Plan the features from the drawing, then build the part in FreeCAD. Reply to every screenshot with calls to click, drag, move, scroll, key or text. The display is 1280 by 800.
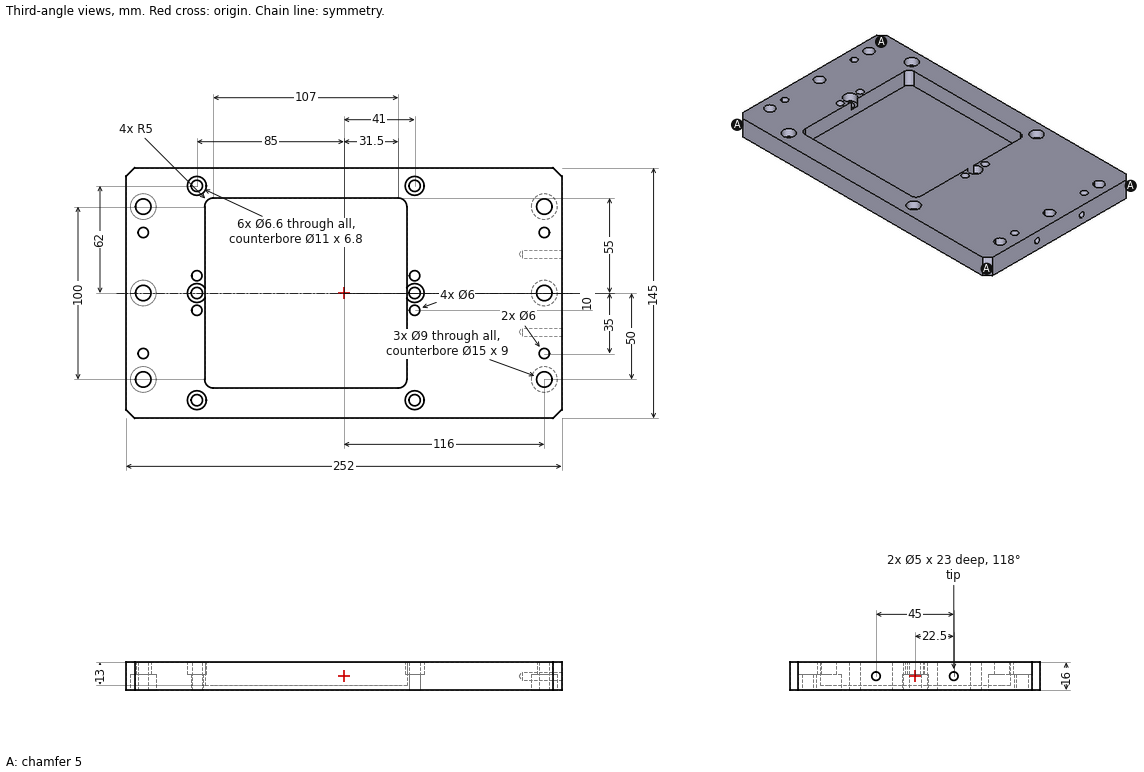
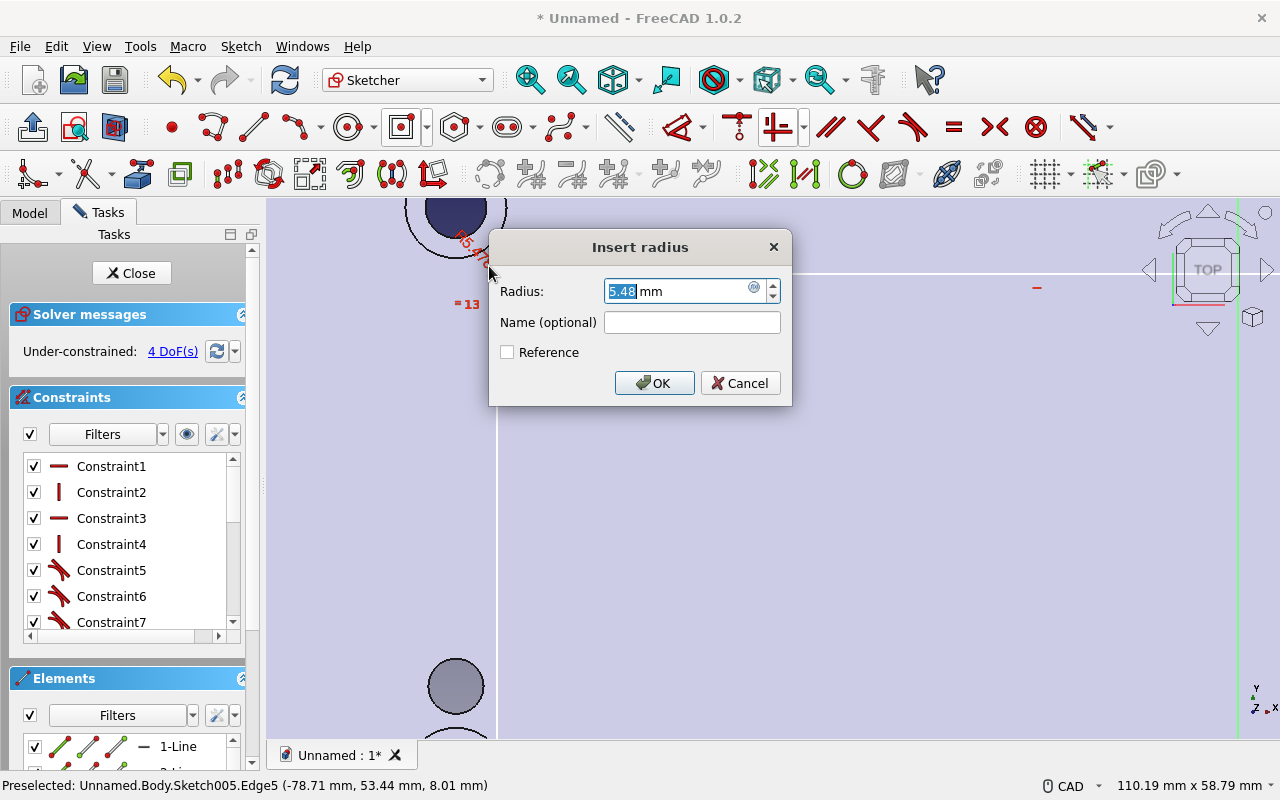
text(5)
key(Return)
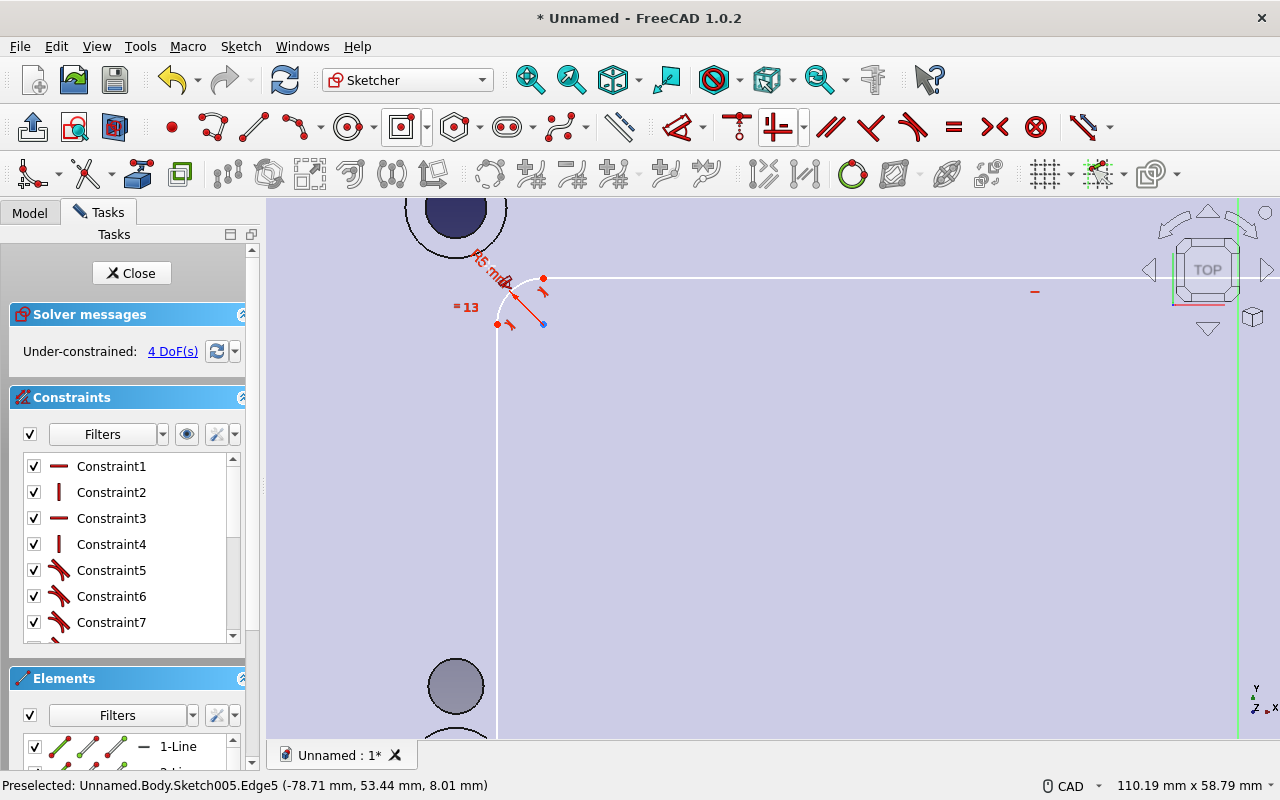
click(838, 278)
click(829, 244)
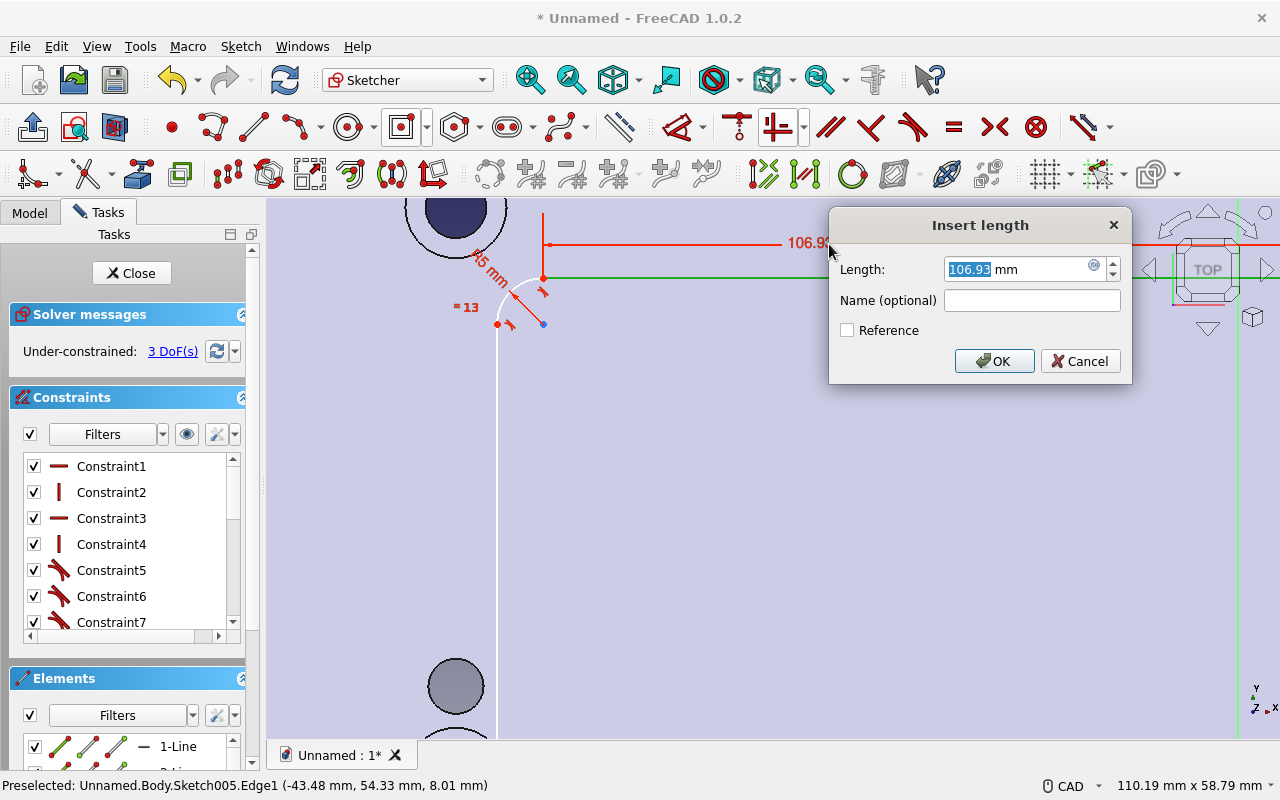
text(107)
key(Return)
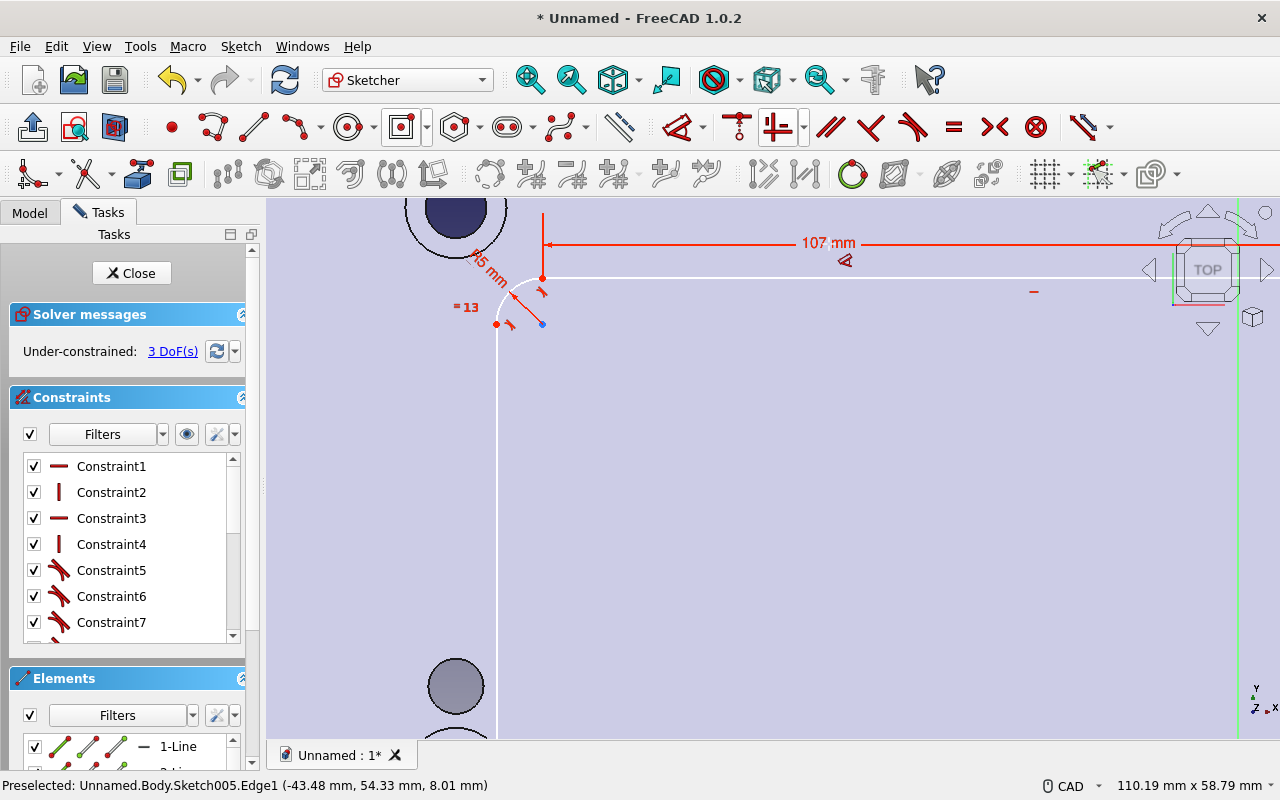
click(497, 599)
click(463, 518)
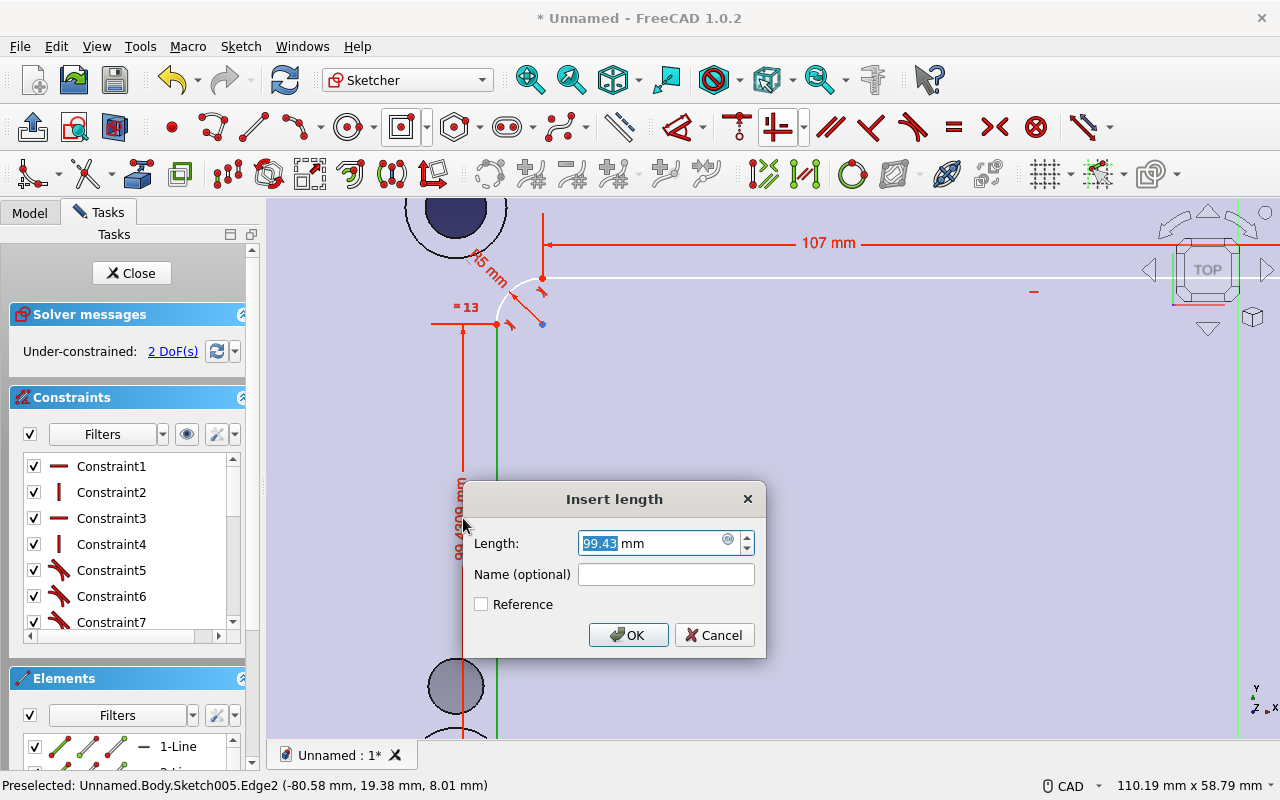
text(100)
key(Return)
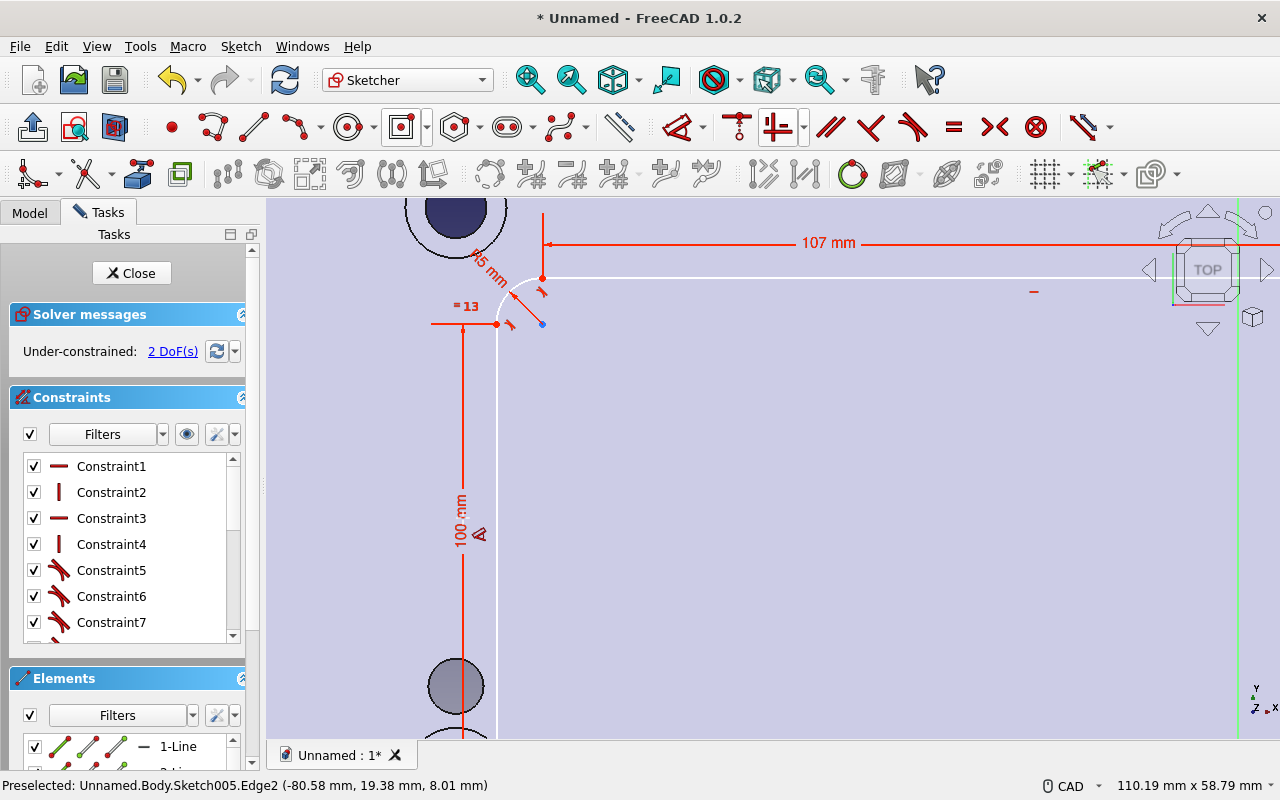
scroll(512, 288, down, 5)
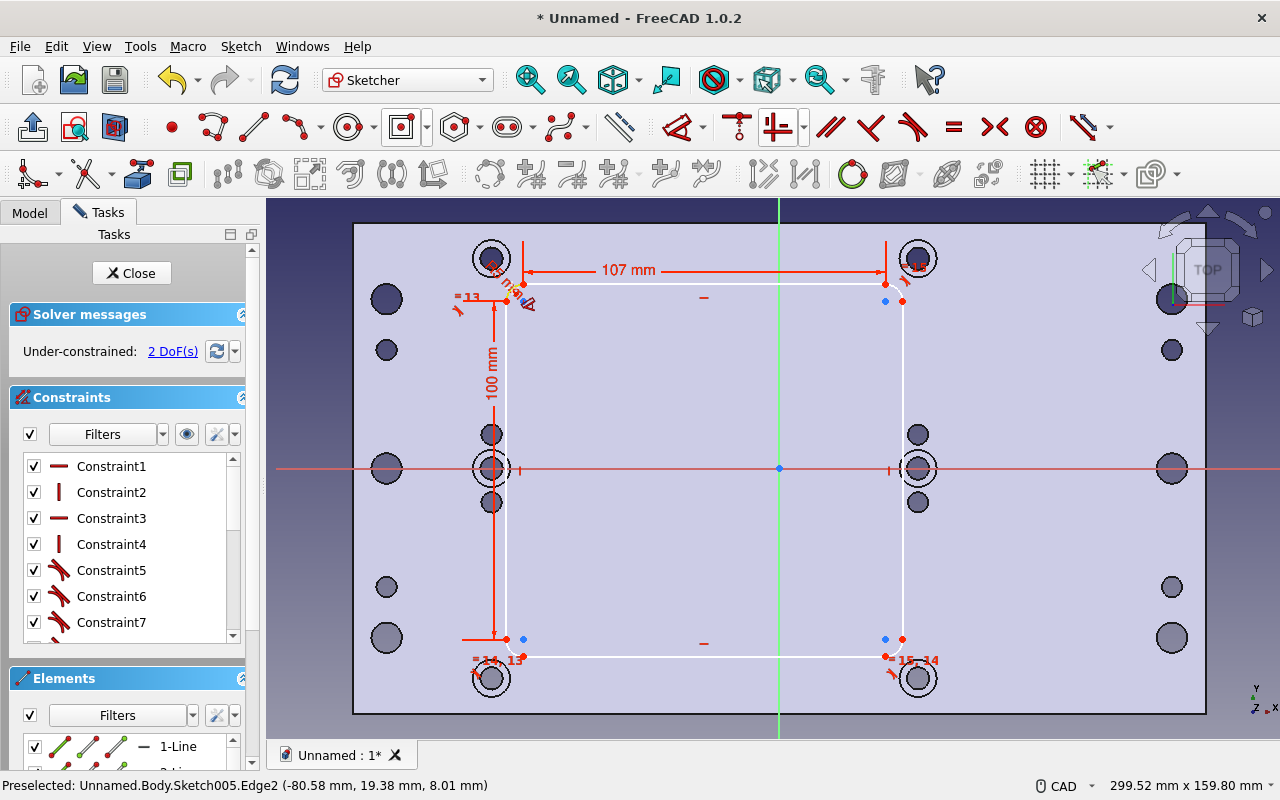
click(886, 284)
click(920, 376)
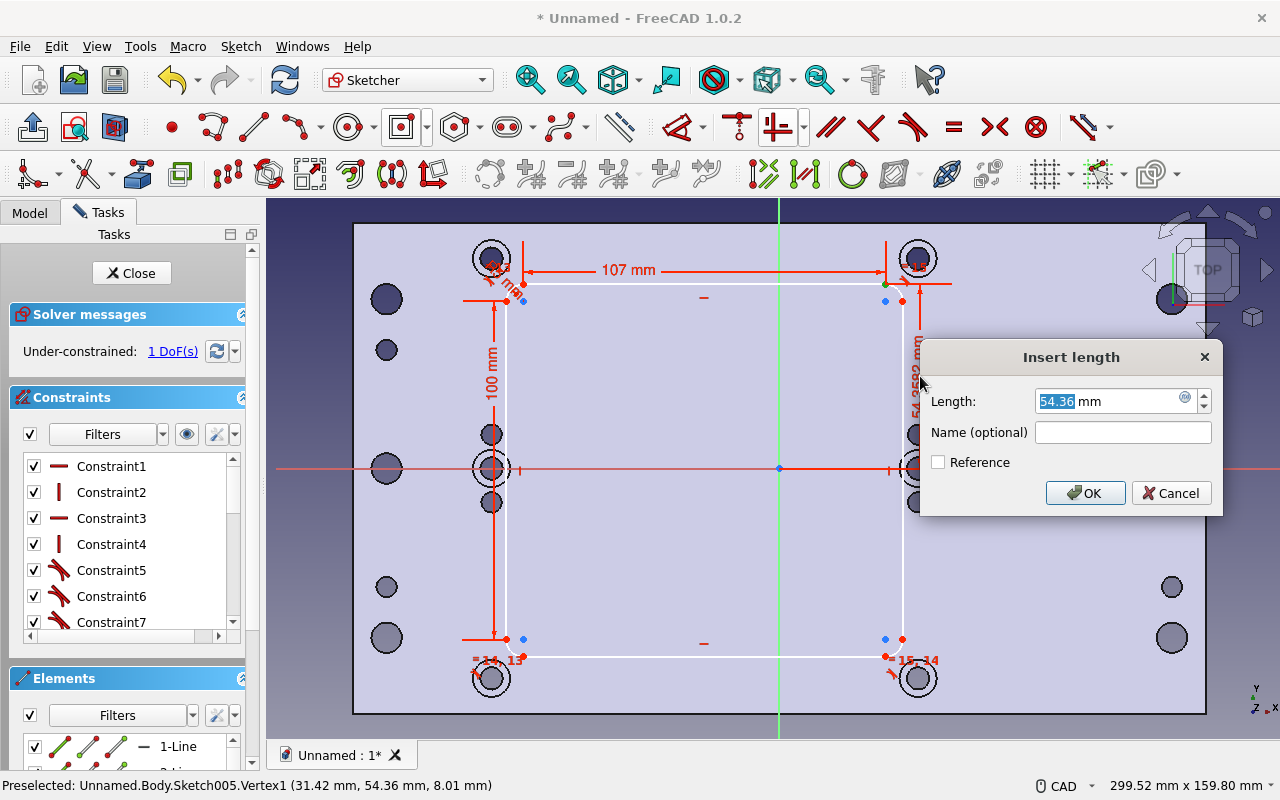
text(55)
key(Return)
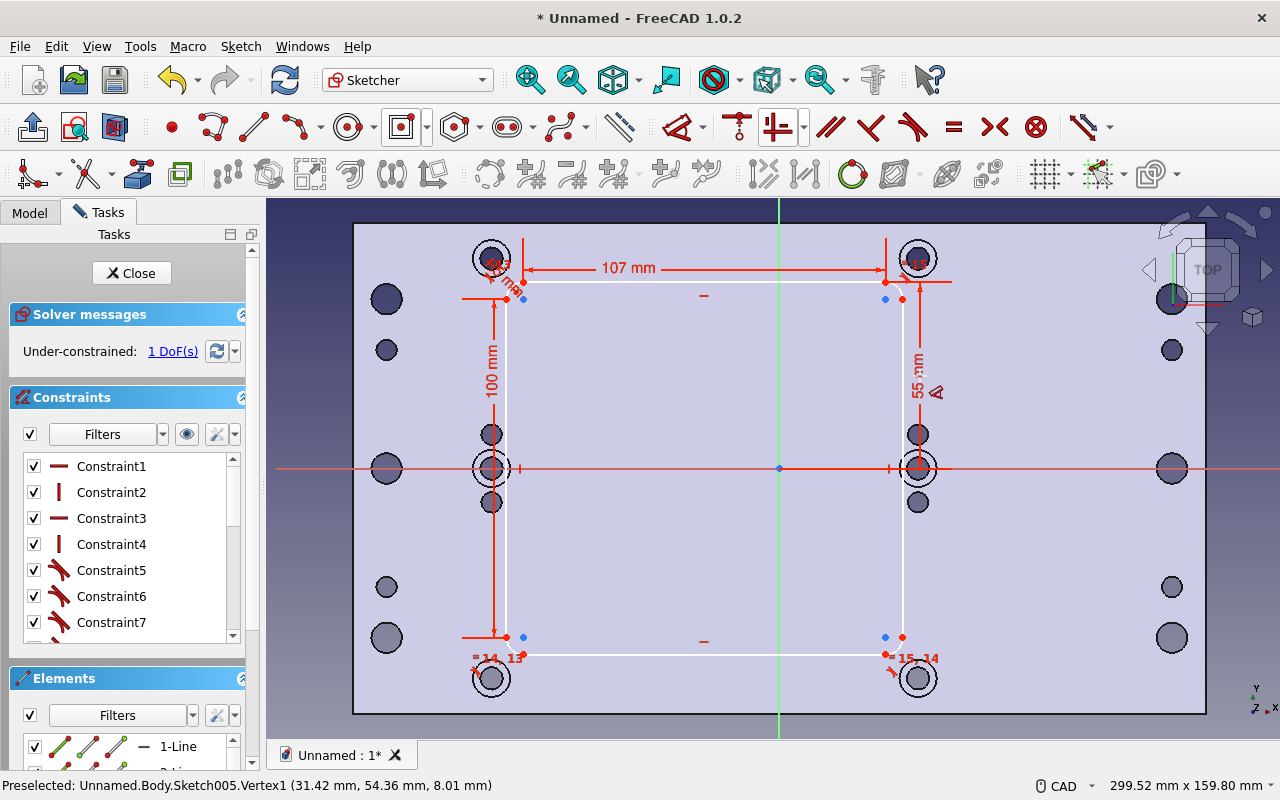
click(886, 282)
click(832, 248)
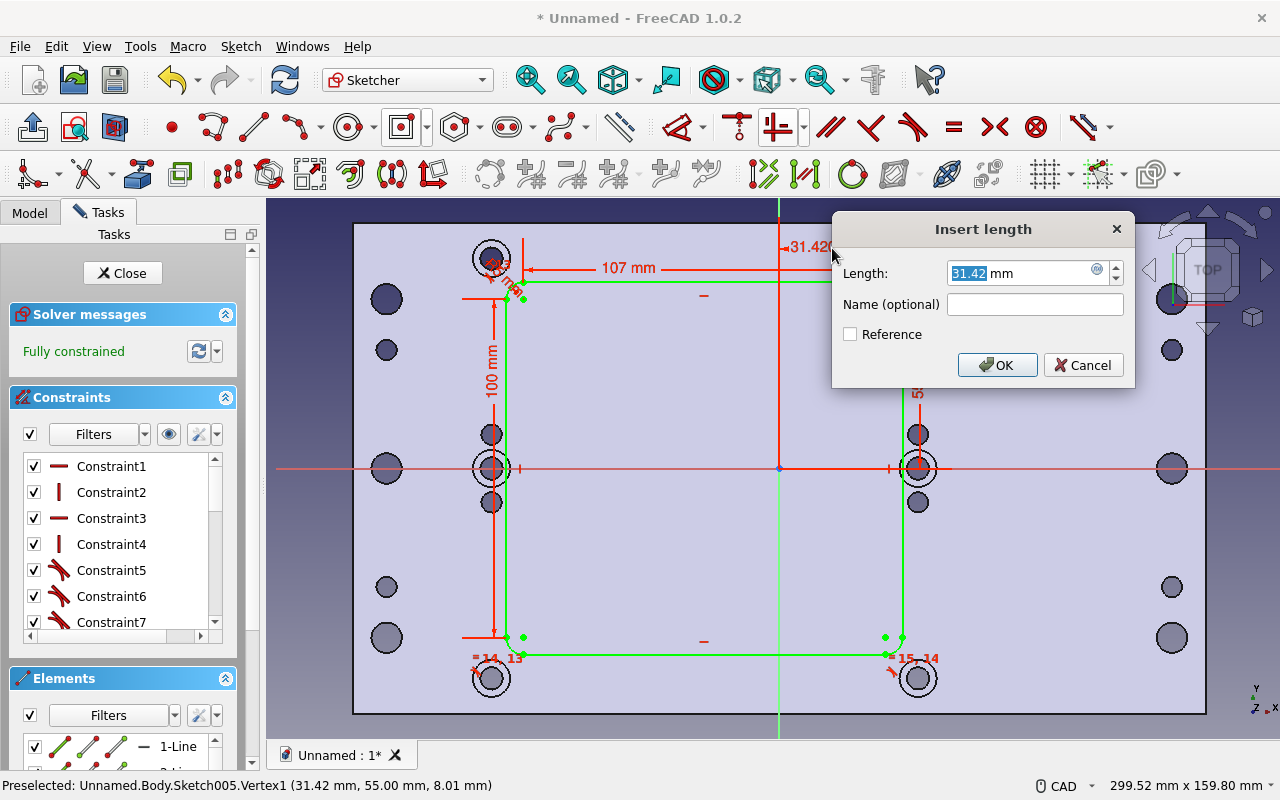
text(31.5)
key(Return)
key(Escape)